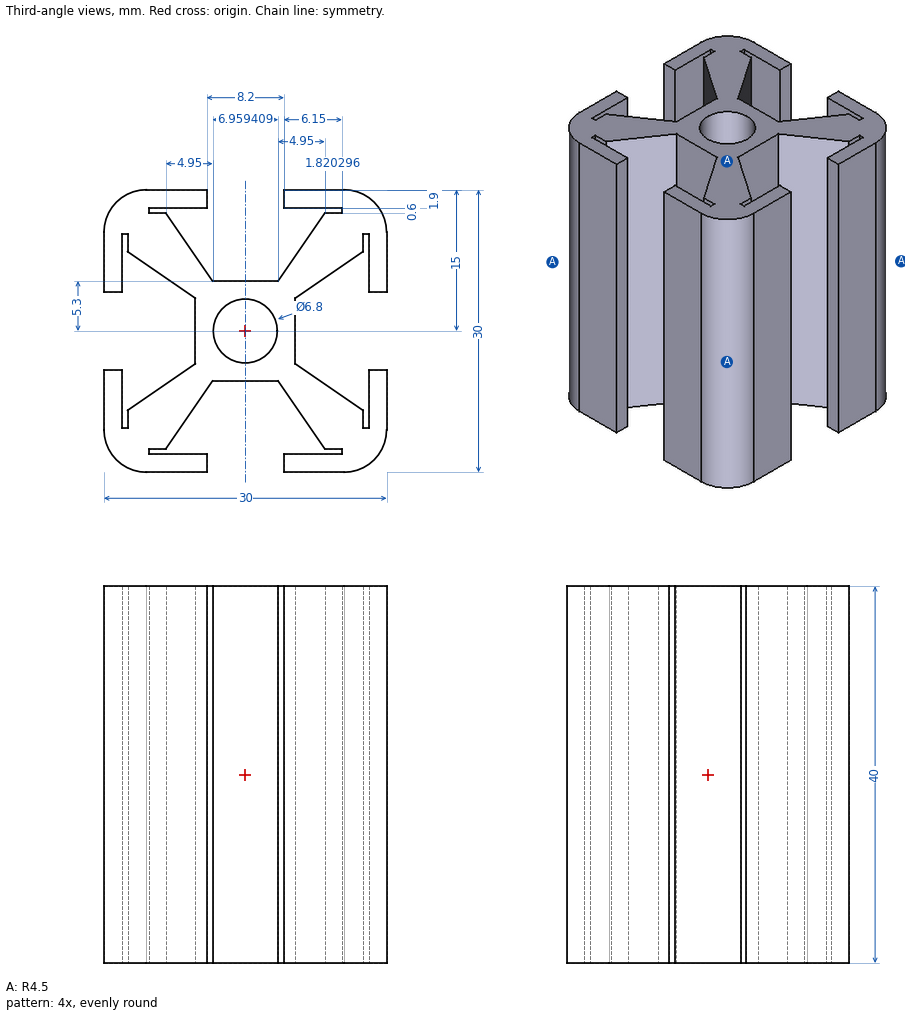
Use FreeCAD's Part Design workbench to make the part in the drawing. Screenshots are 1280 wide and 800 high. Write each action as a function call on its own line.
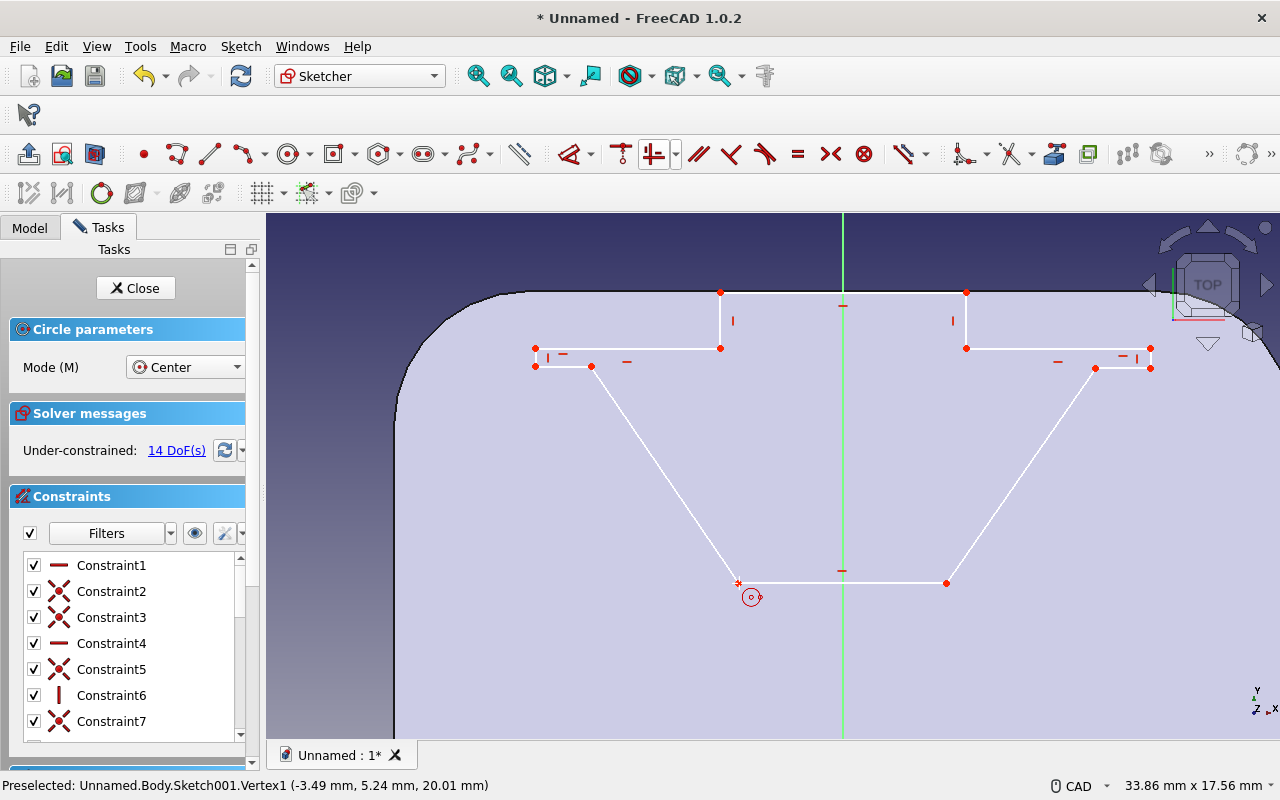
scroll(536, 366, down, 3)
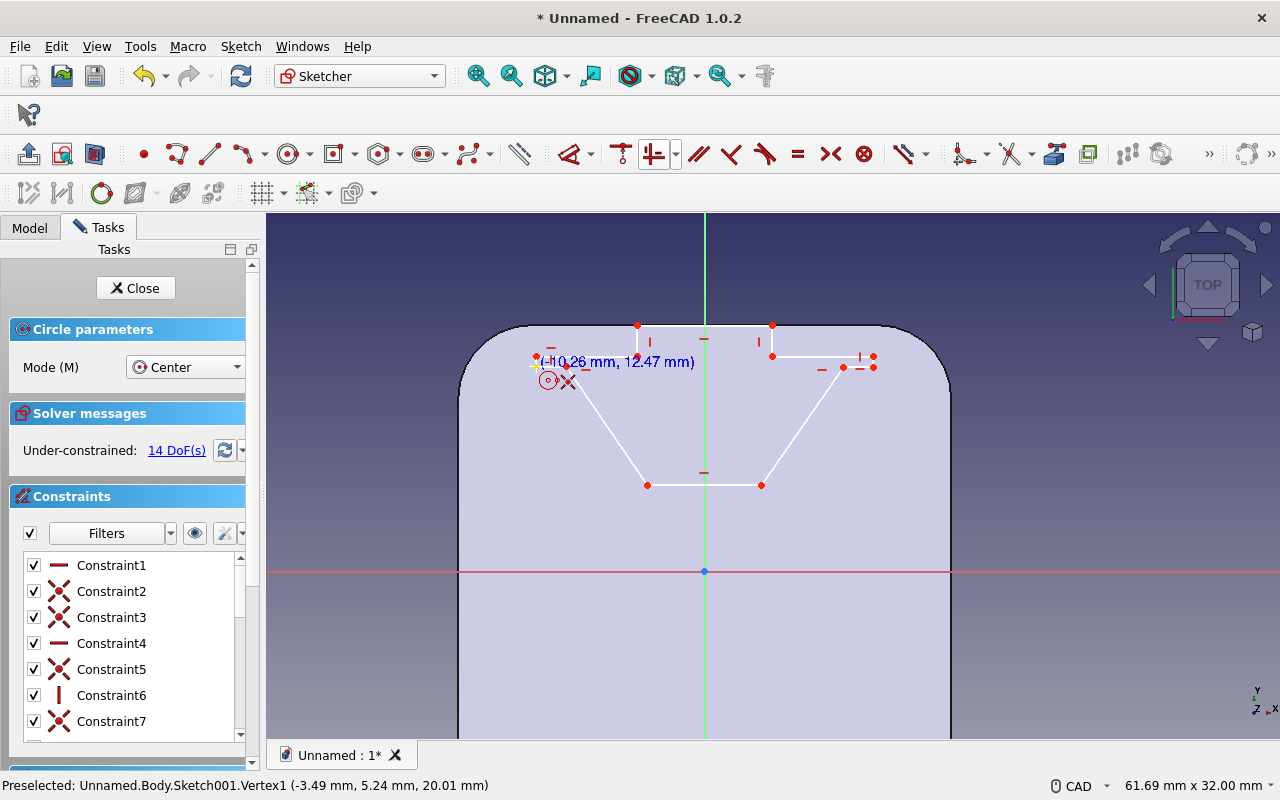
click(705, 572)
move(744, 532)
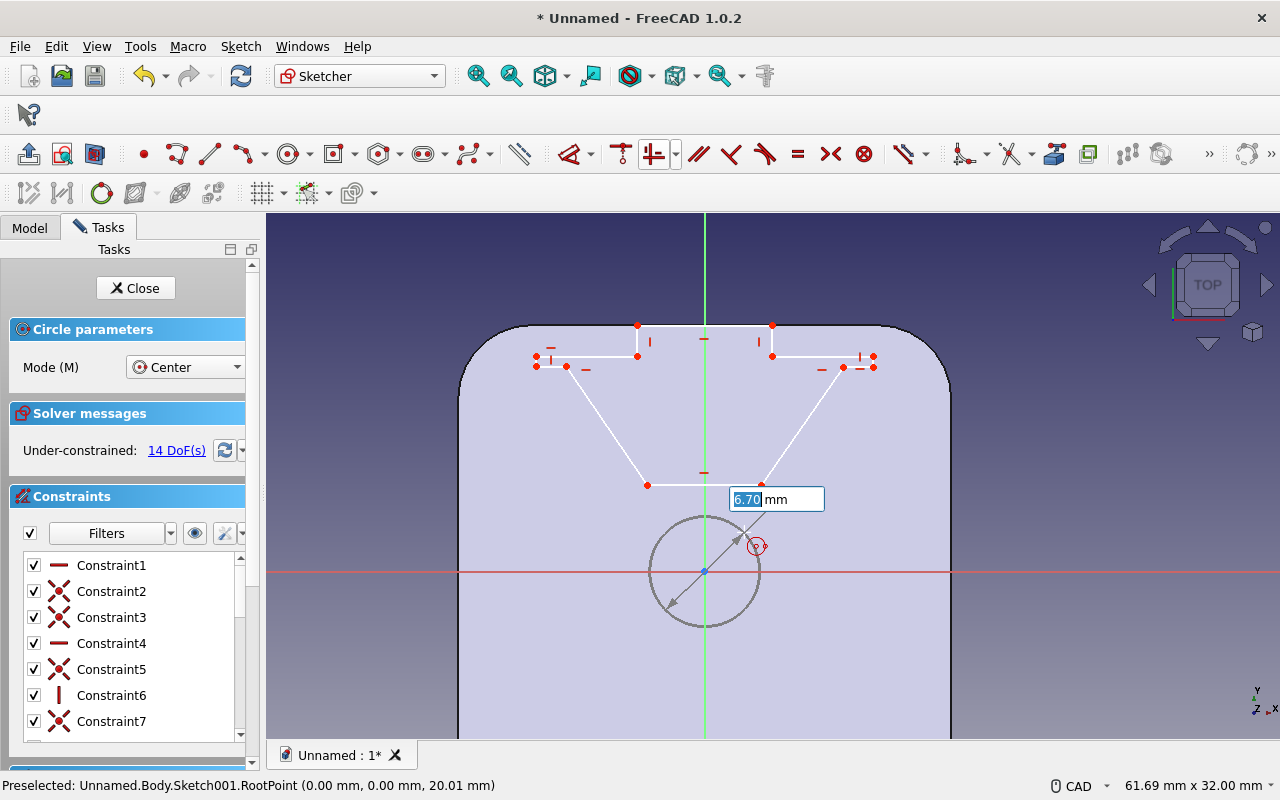
text(6.8)
key(Return)
key(Escape)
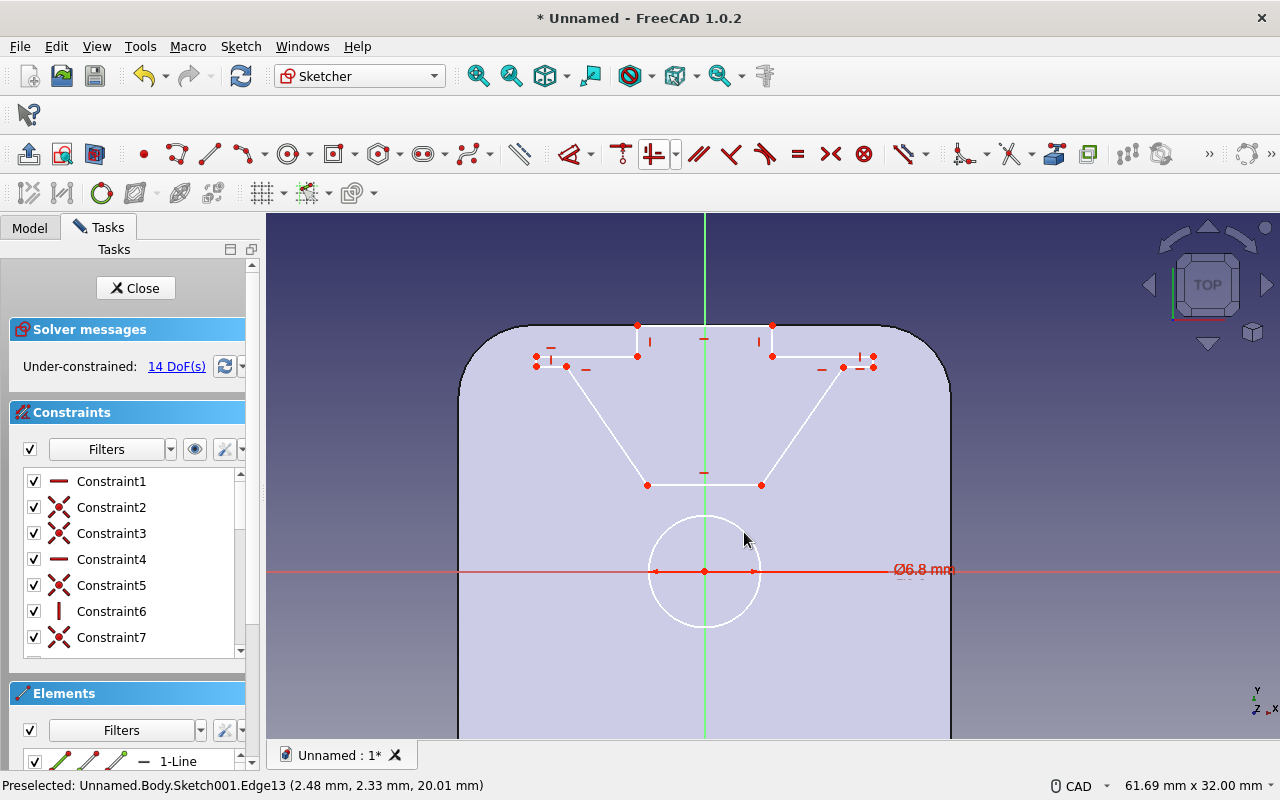
click(772, 357)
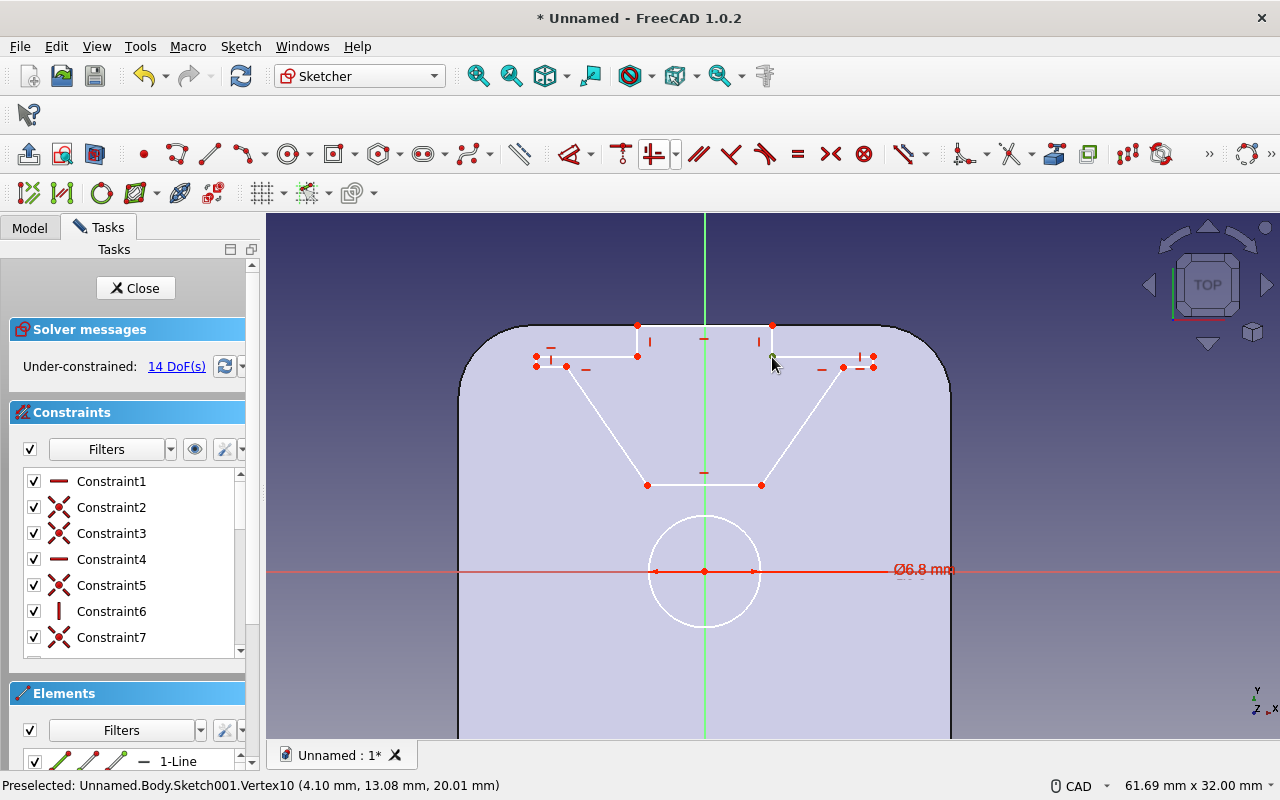
click(637, 357)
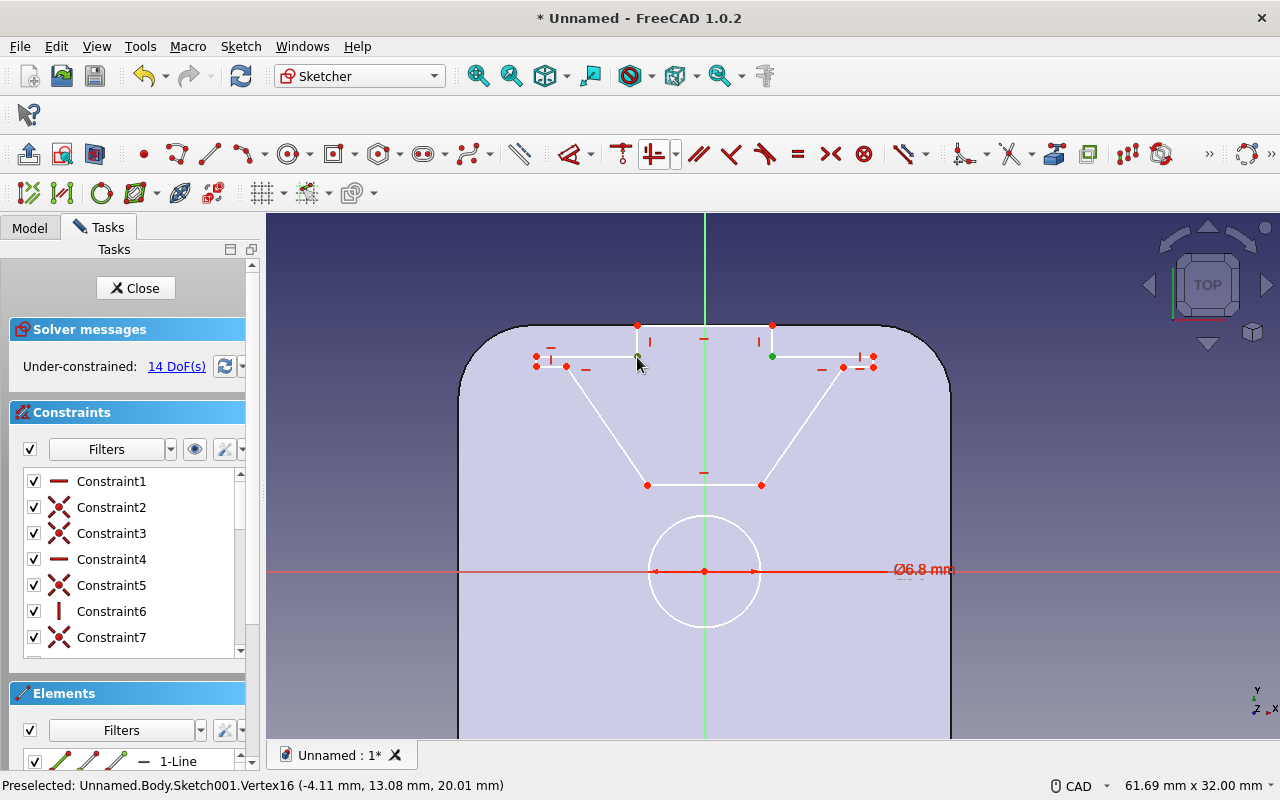
click(705, 677)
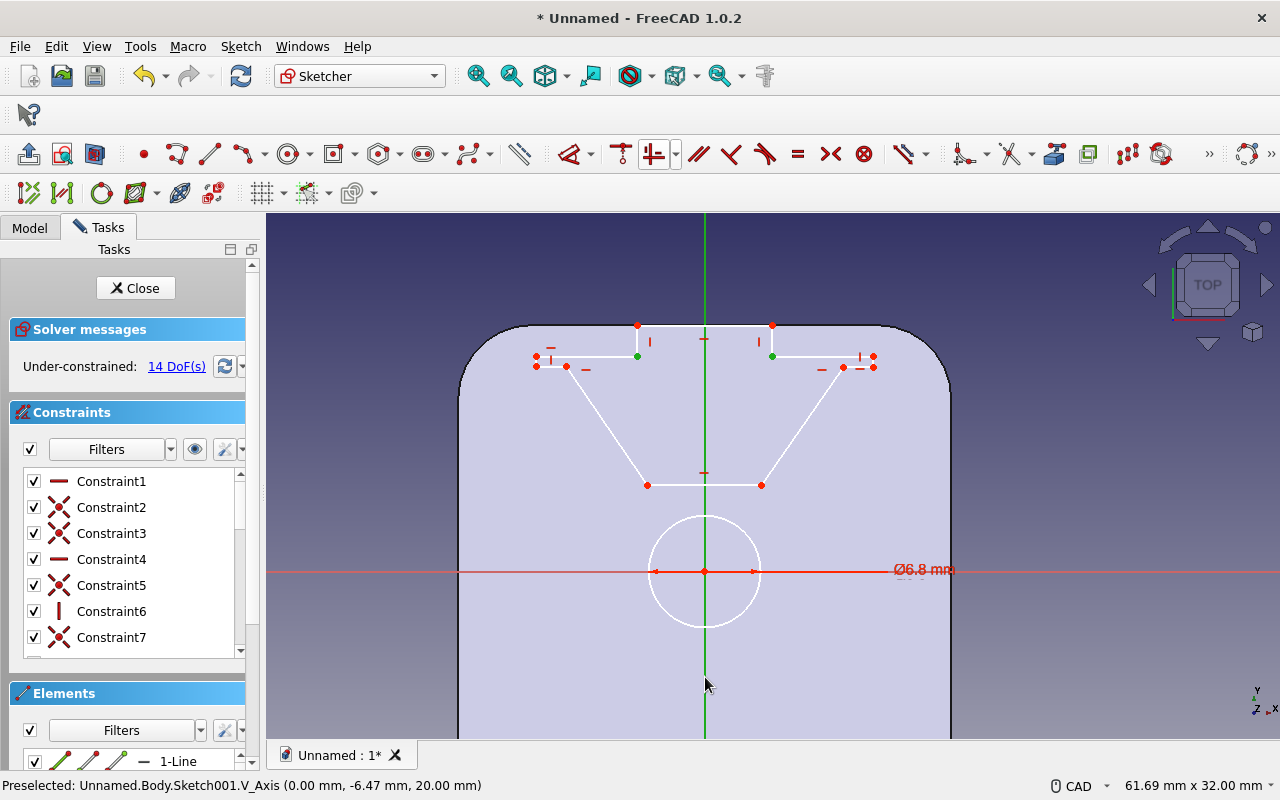
click(831, 154)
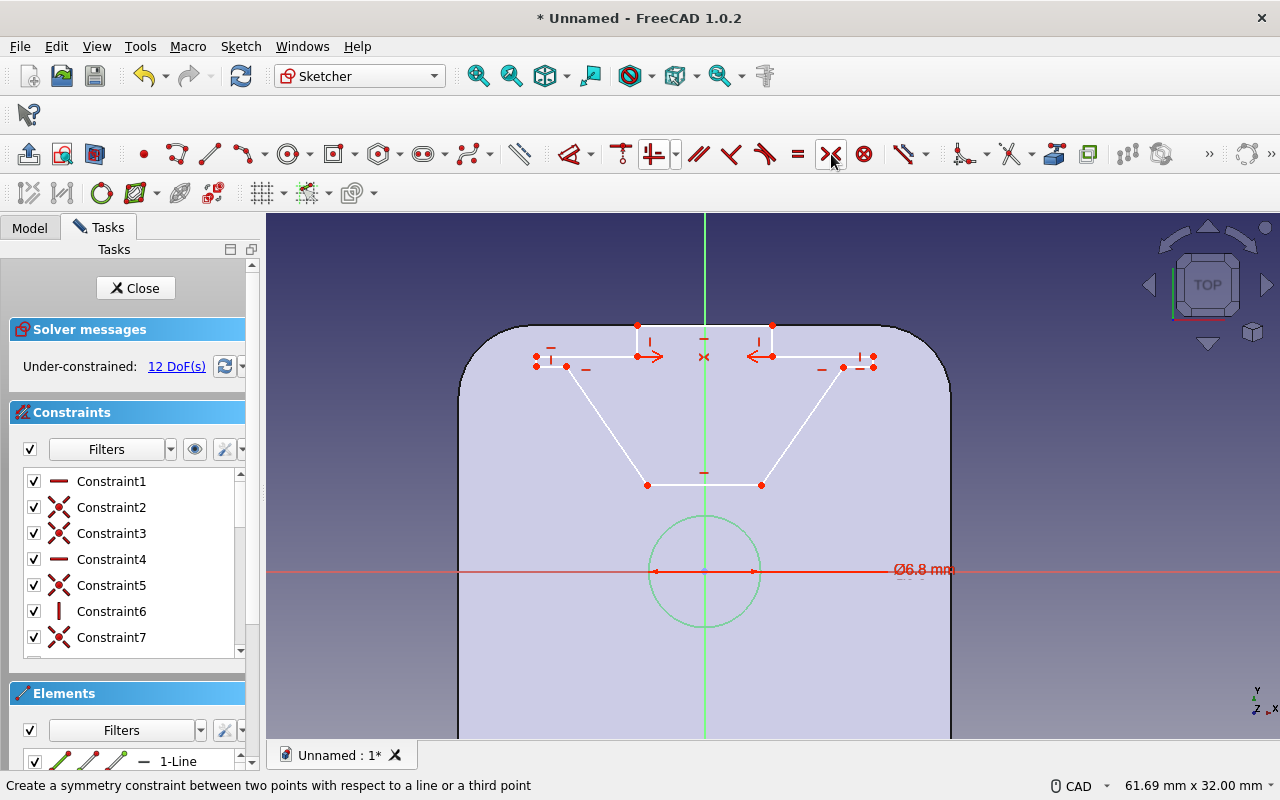
click(873, 367)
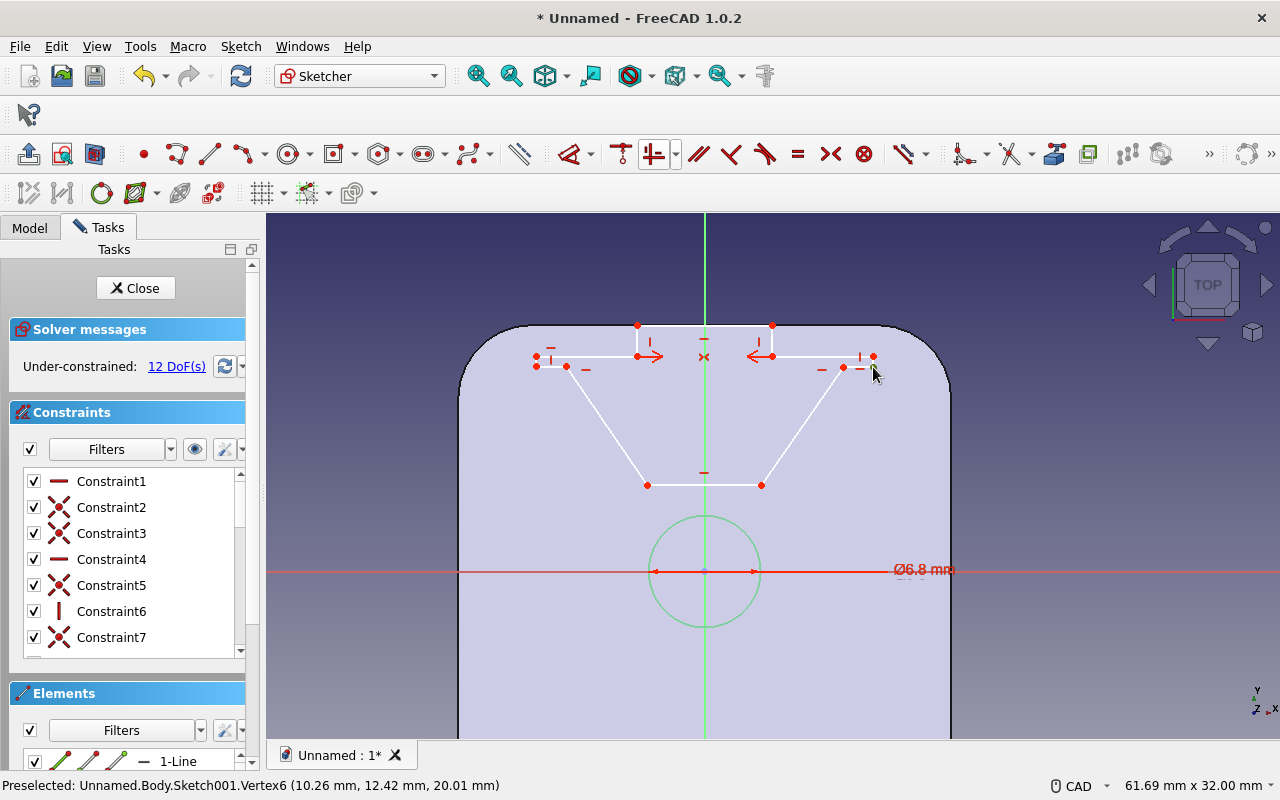
click(536, 367)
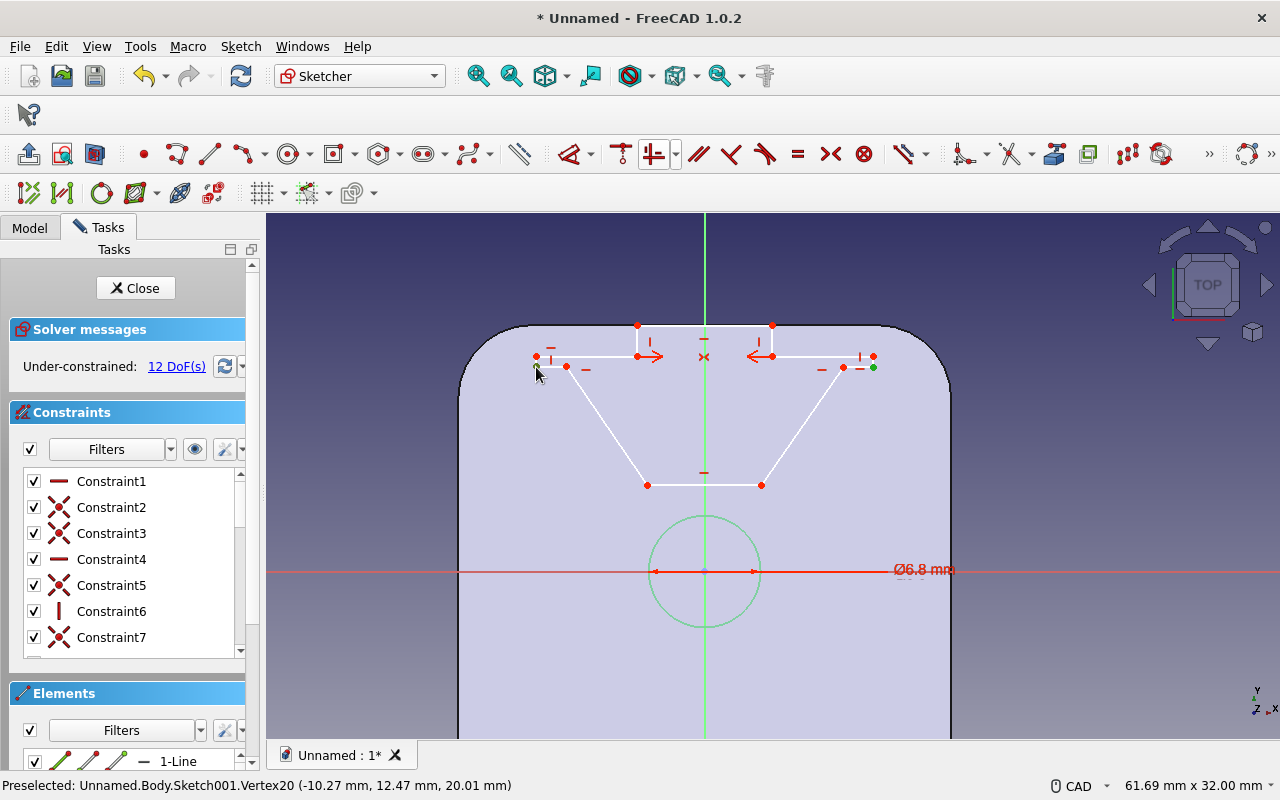
click(705, 677)